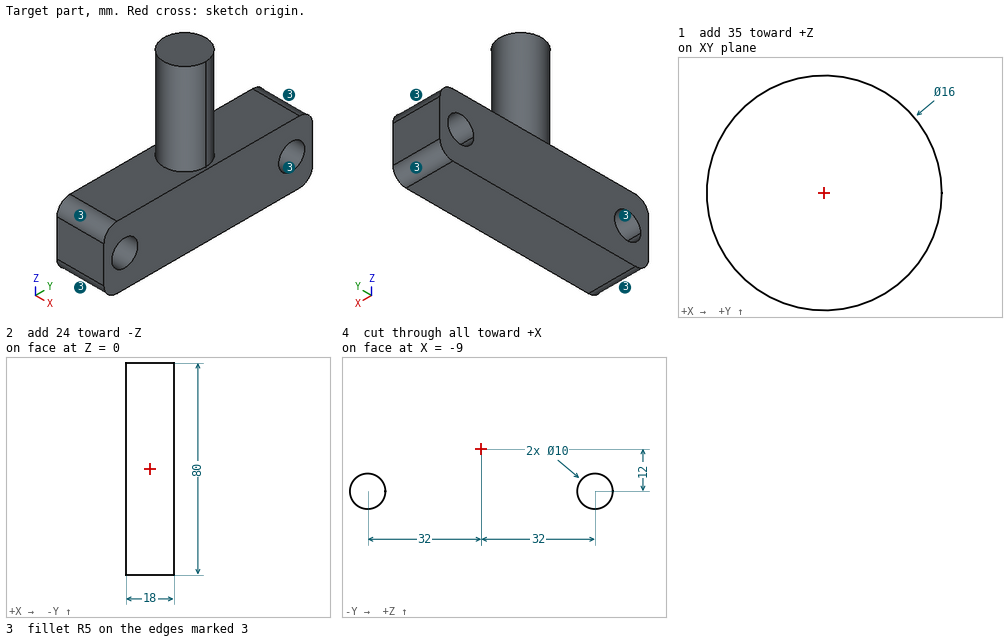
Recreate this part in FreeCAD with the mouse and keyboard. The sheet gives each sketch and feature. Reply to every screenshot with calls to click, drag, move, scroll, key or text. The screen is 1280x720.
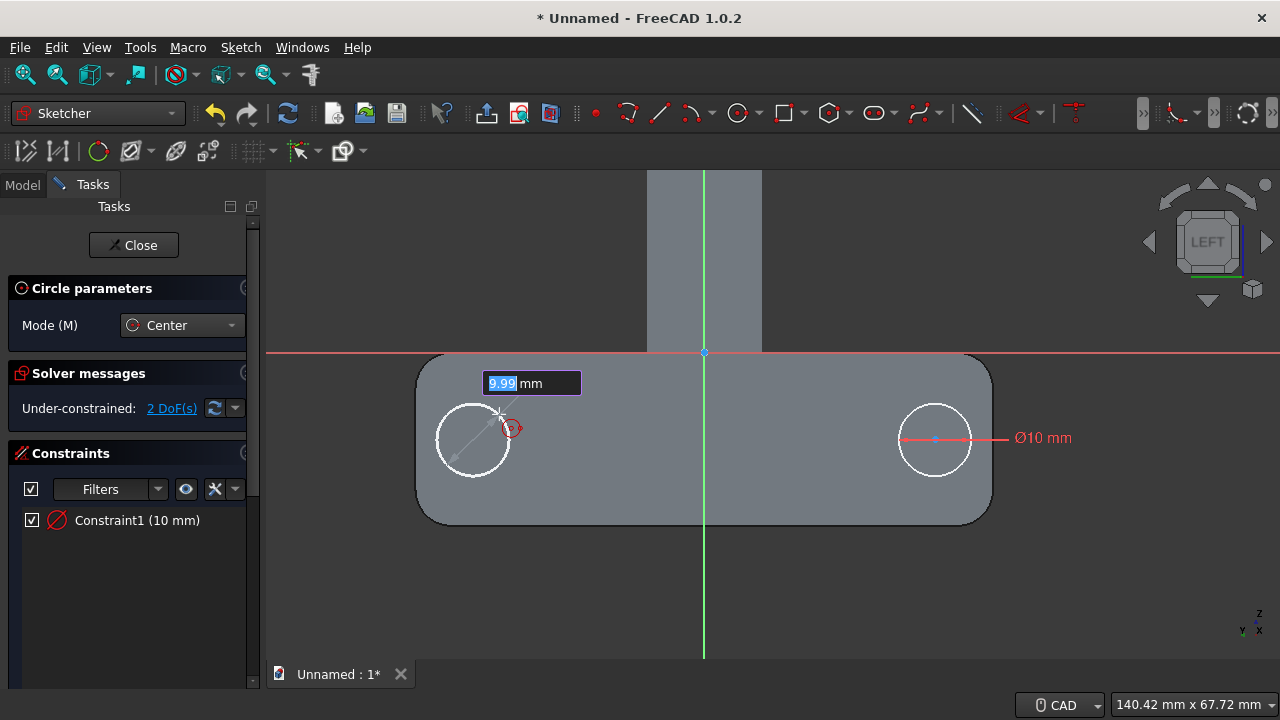
text(10)
key(Return)
key(Escape)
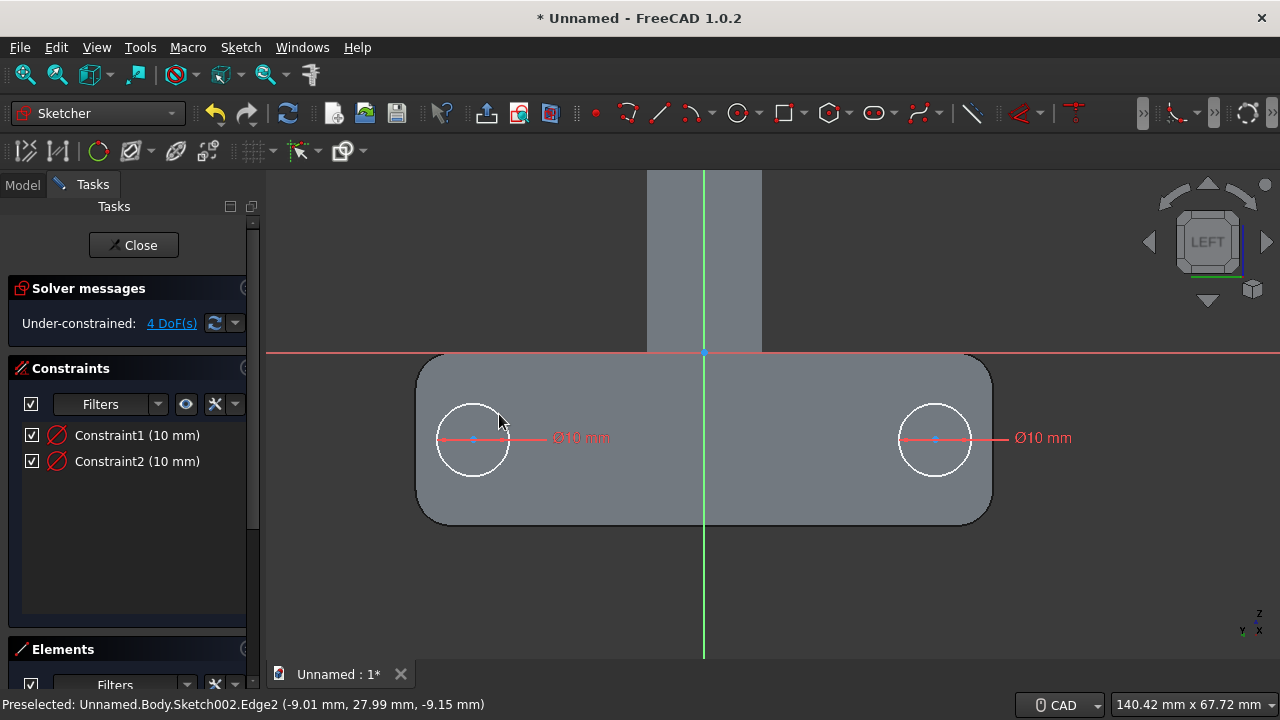
click(935, 440)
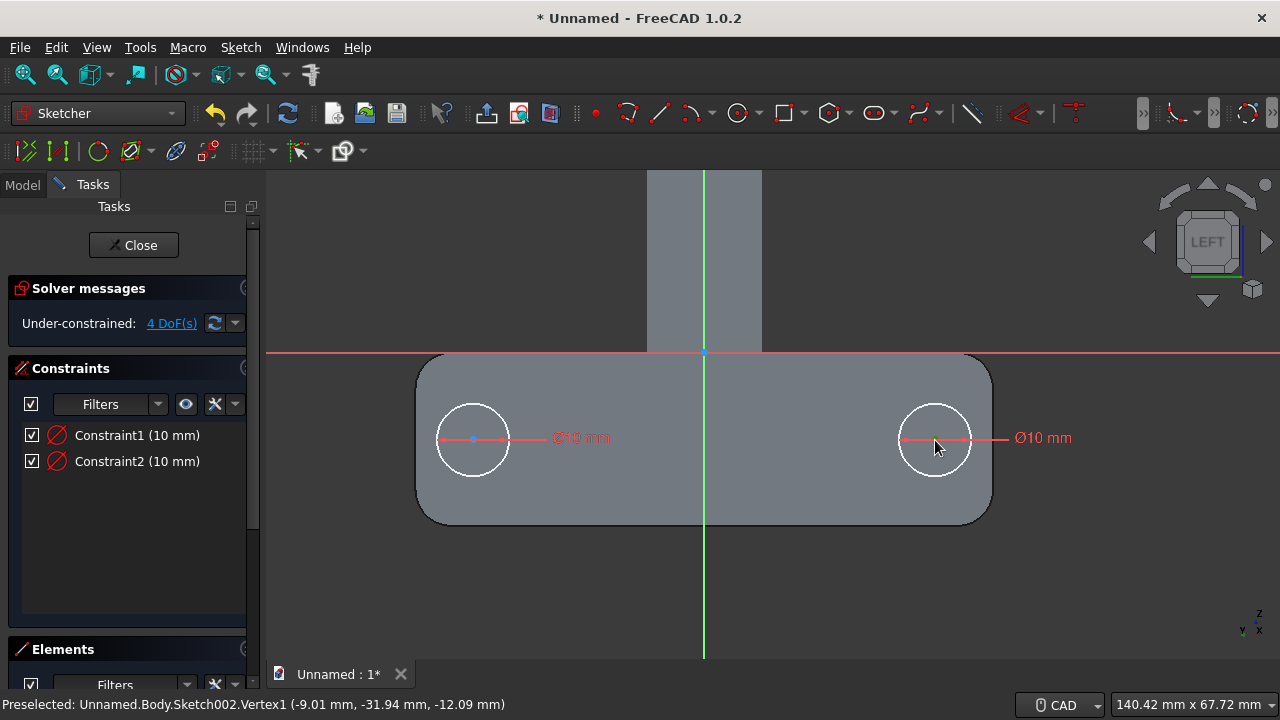
click(473, 440)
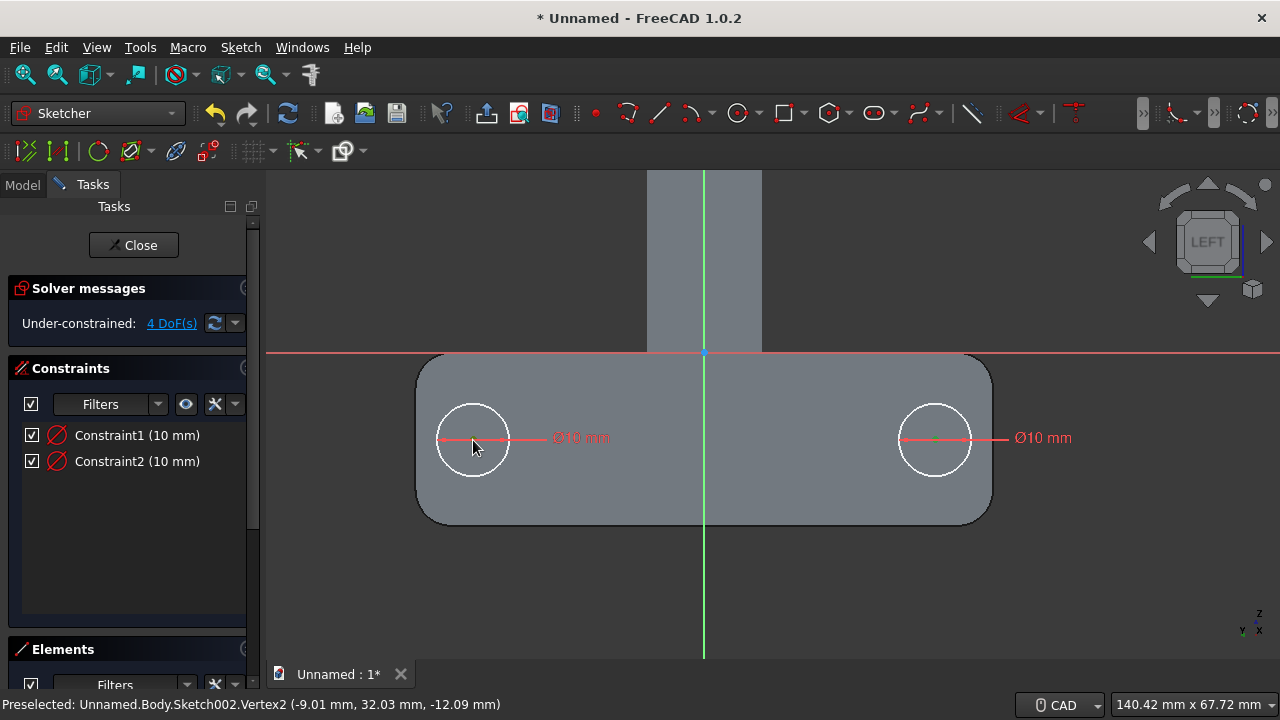
key(h)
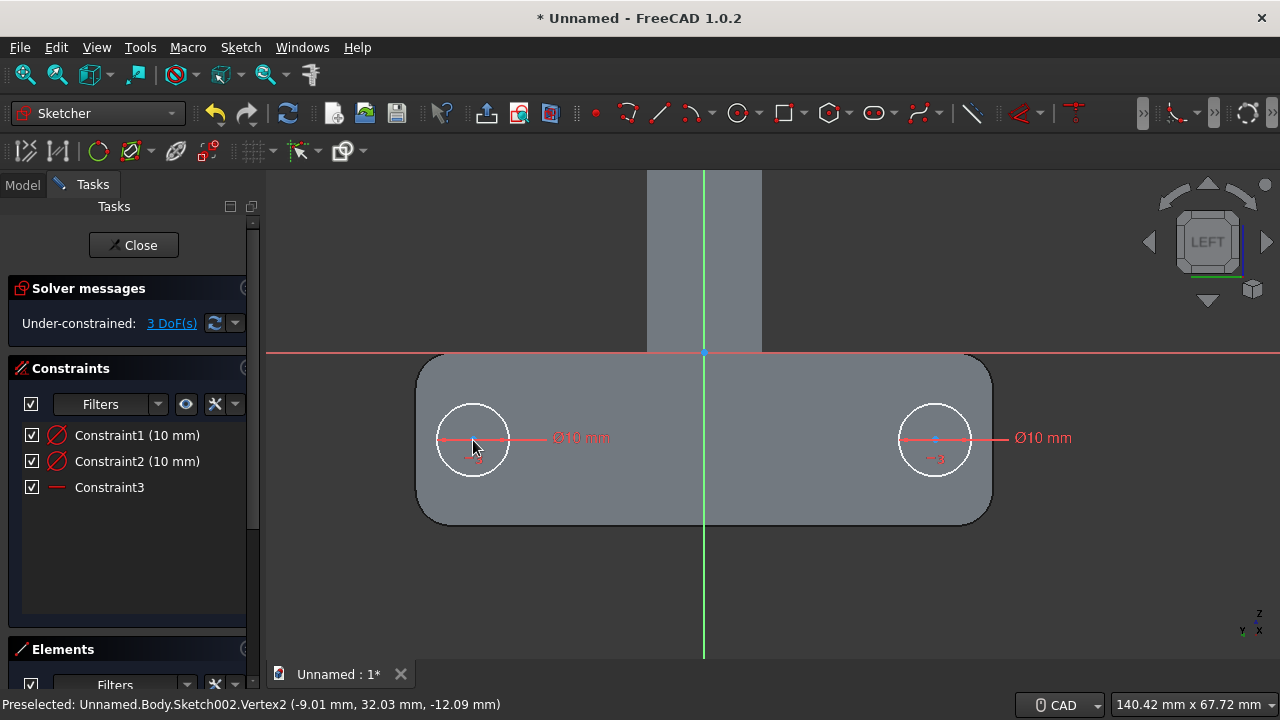
click(1020, 114)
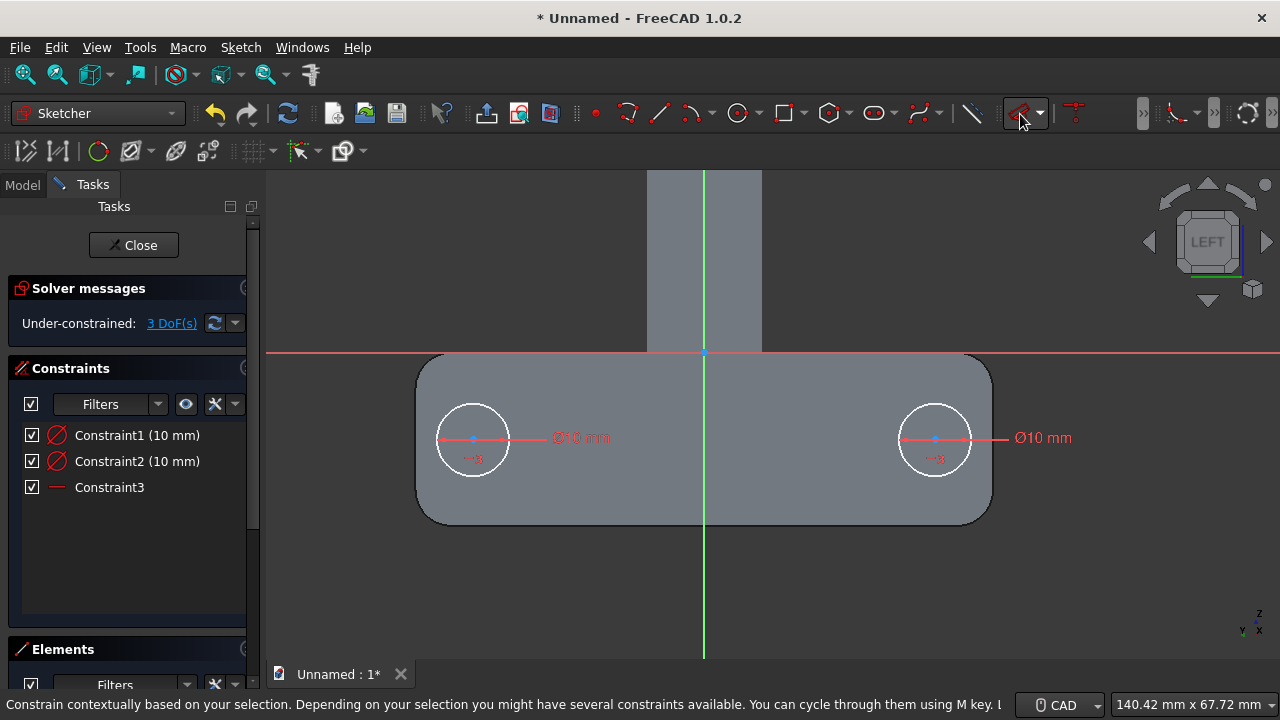
click(935, 440)
click(820, 319)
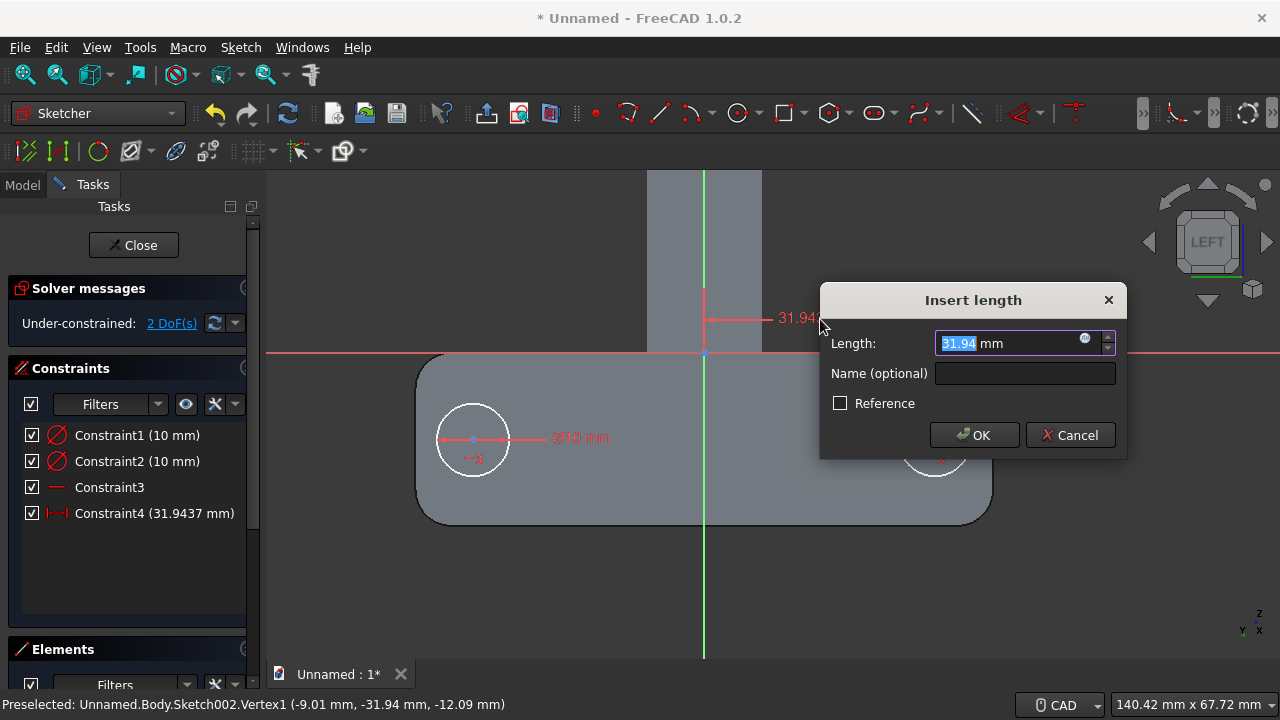
text(32)
key(Return)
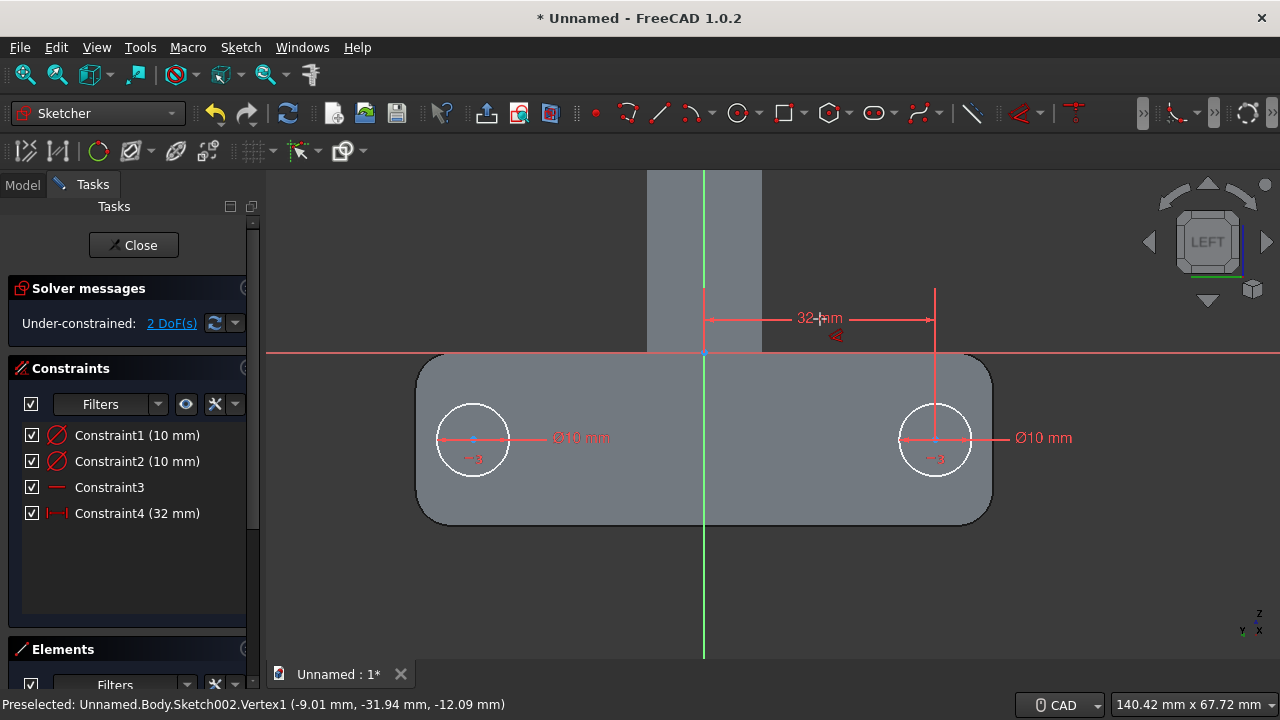
click(935, 440)
click(969, 396)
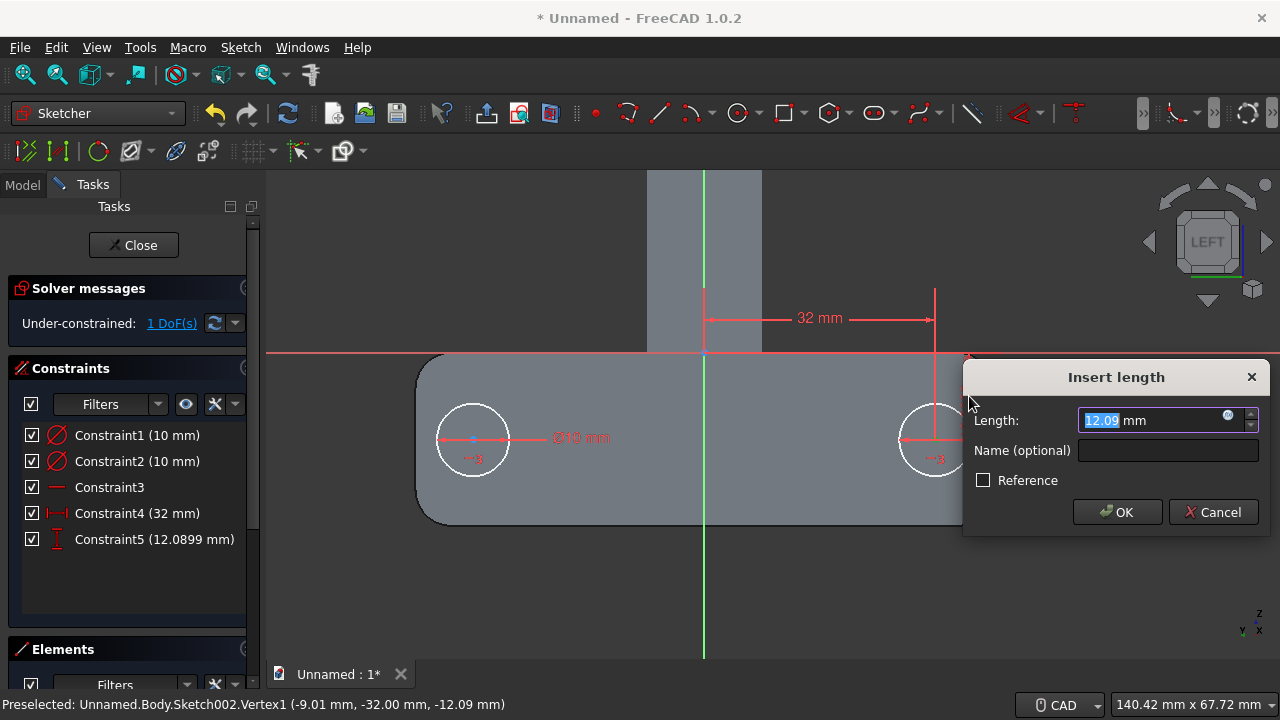
text(12)
key(Return)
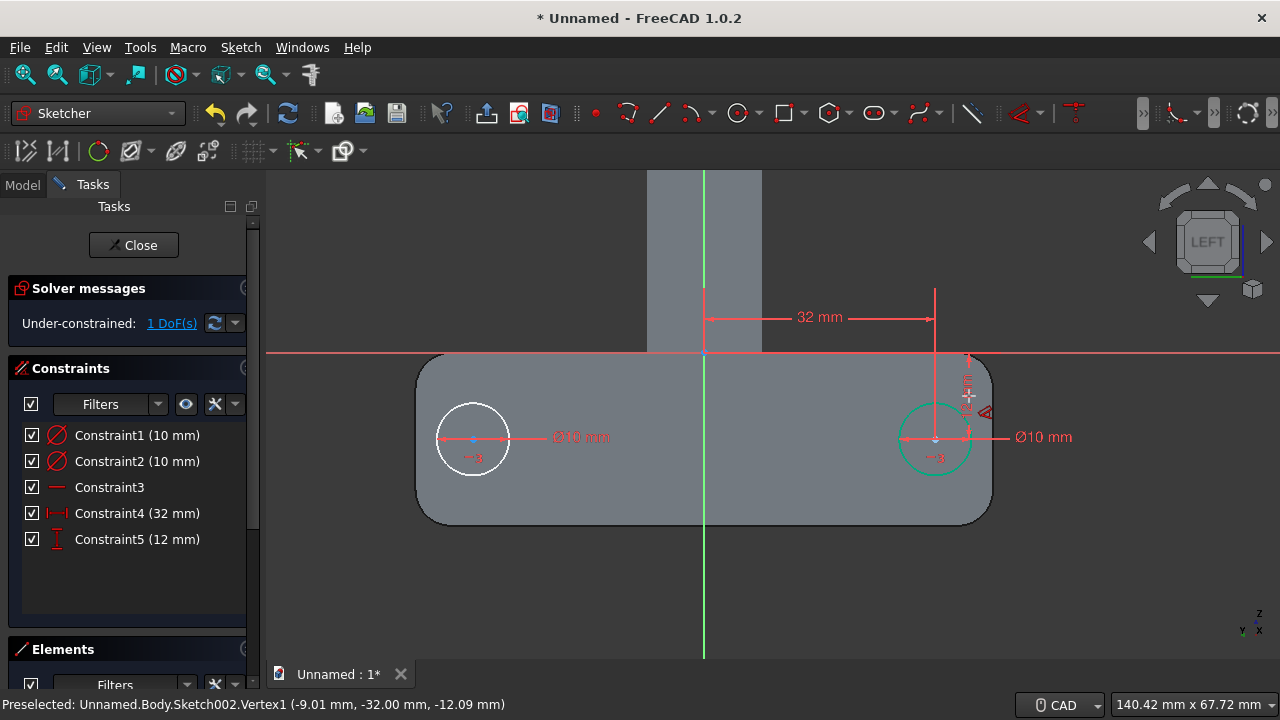
click(473, 439)
click(589, 319)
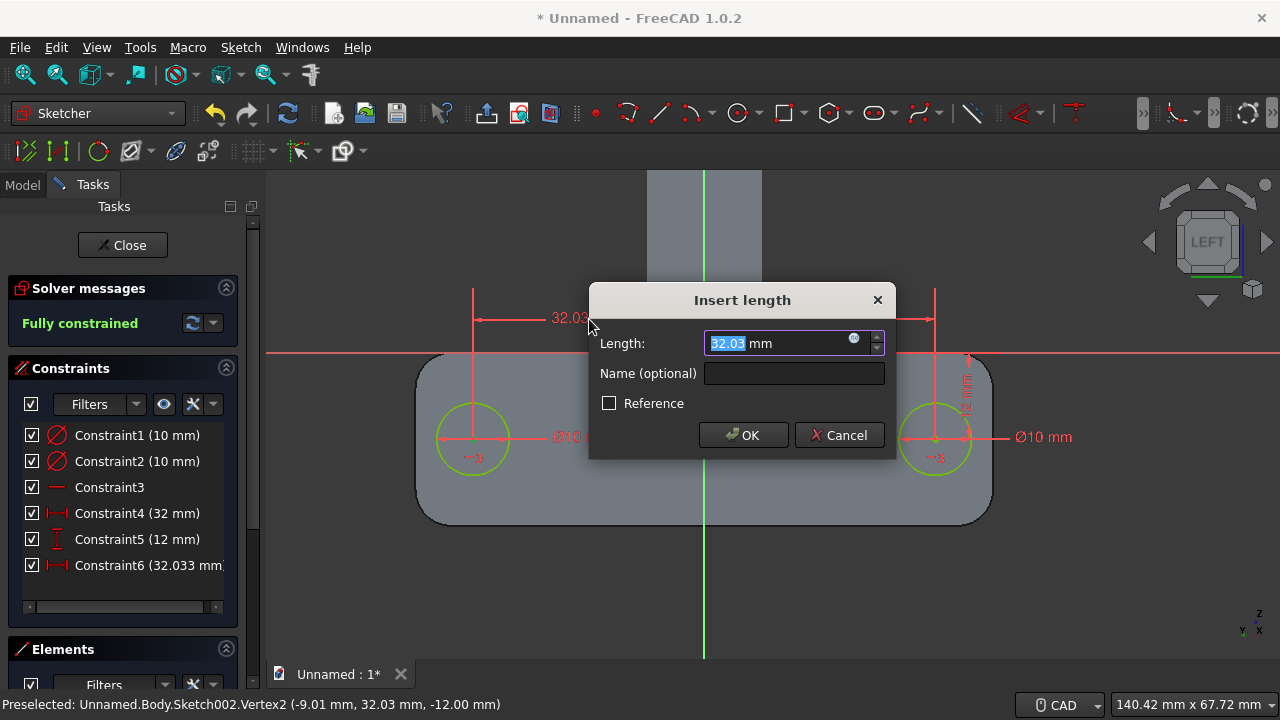
text(32)
key(Return)
key(Escape)